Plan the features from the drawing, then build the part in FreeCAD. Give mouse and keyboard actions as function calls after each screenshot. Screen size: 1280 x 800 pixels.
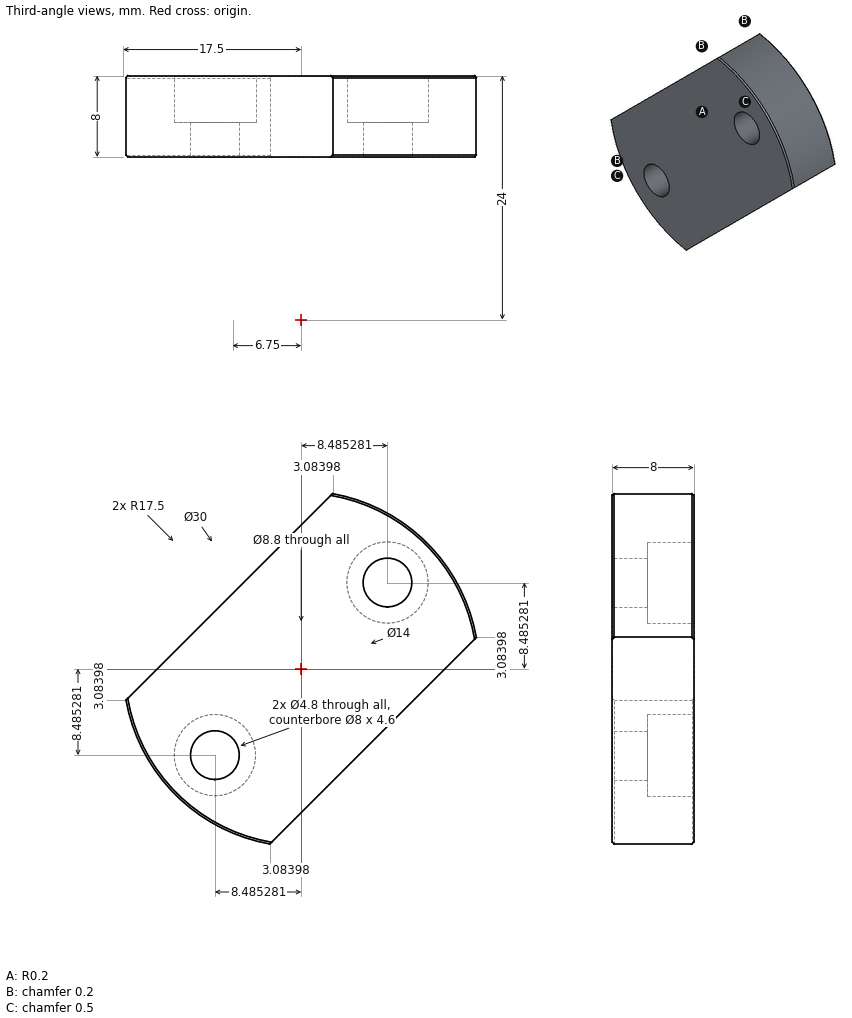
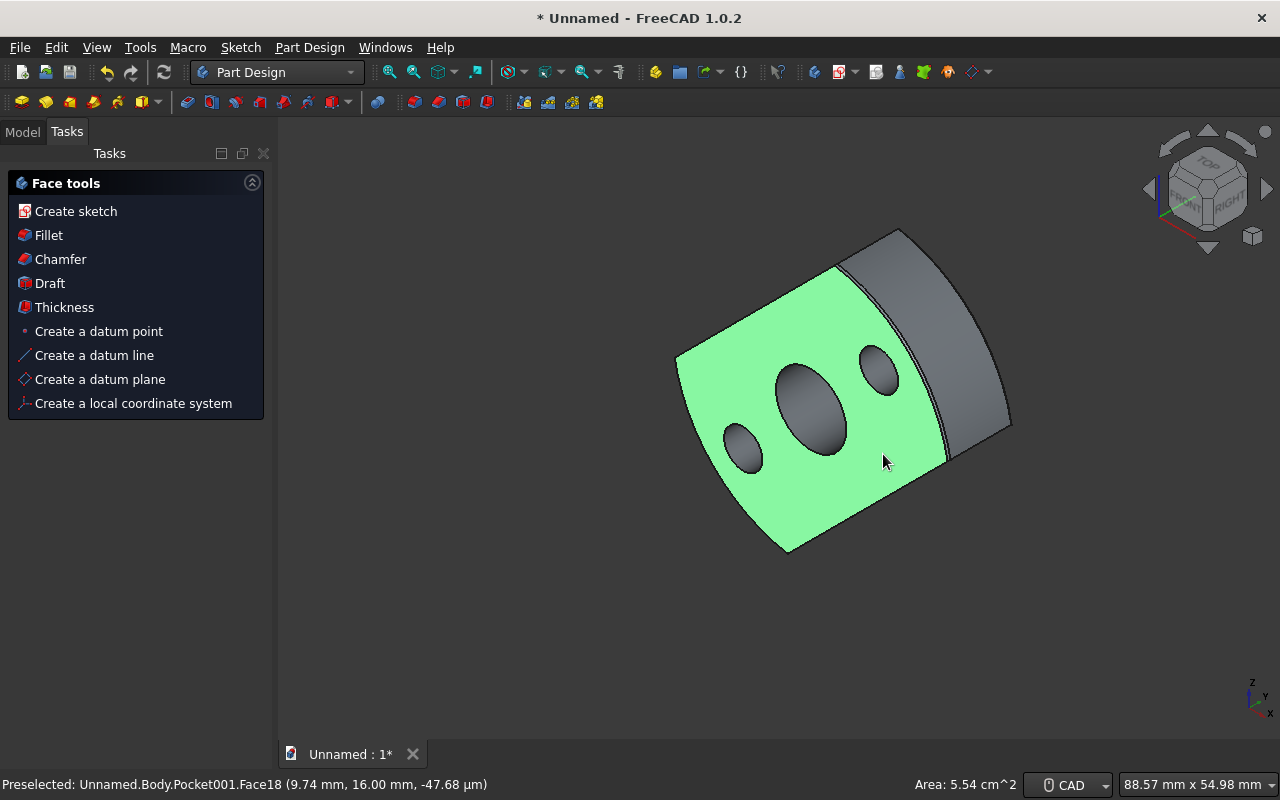
click(840, 72)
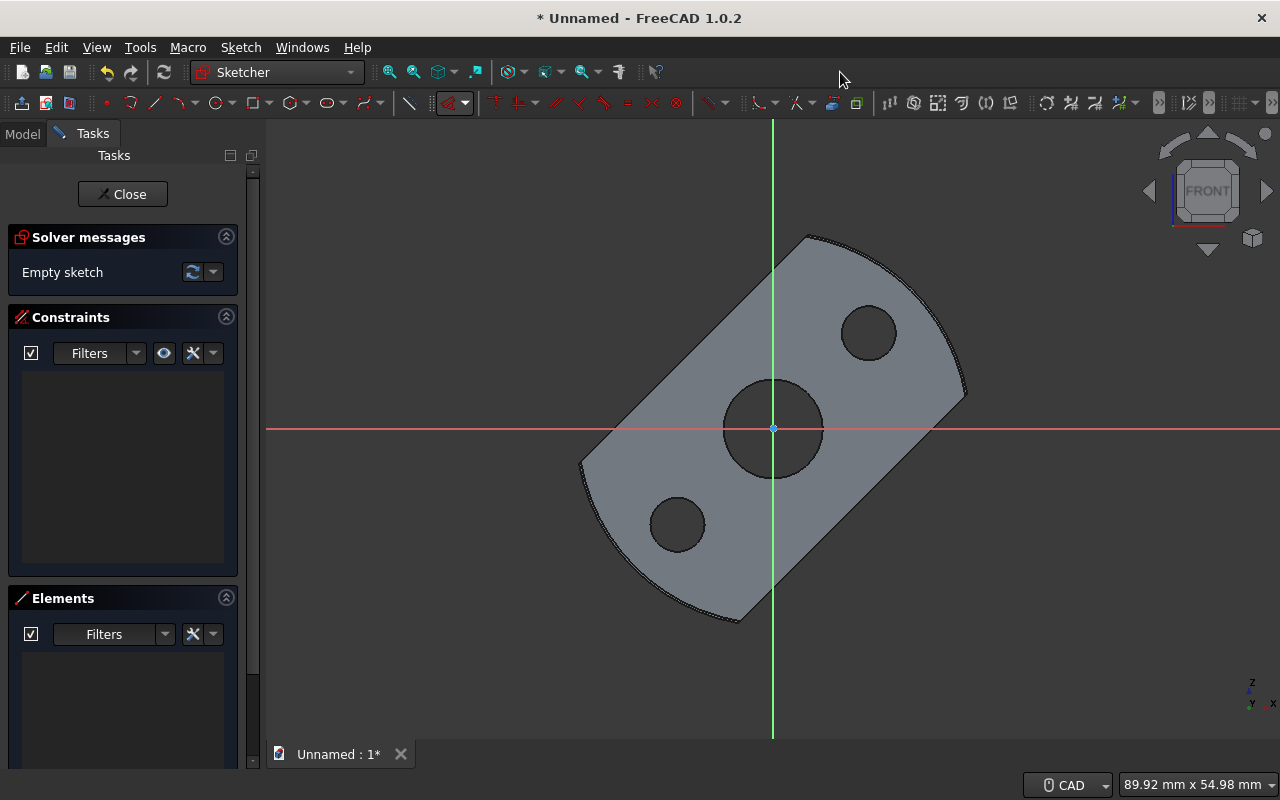
scroll(813, 429, up, 5)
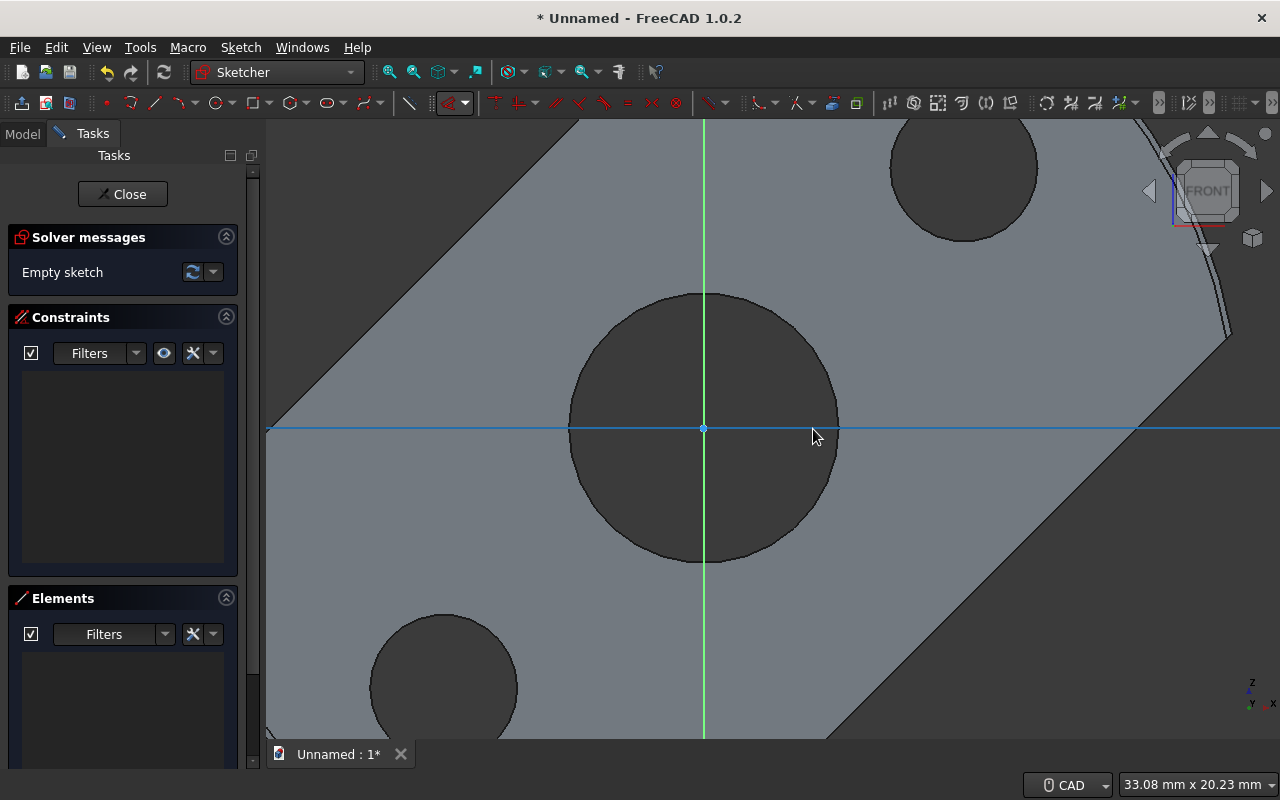
click(216, 104)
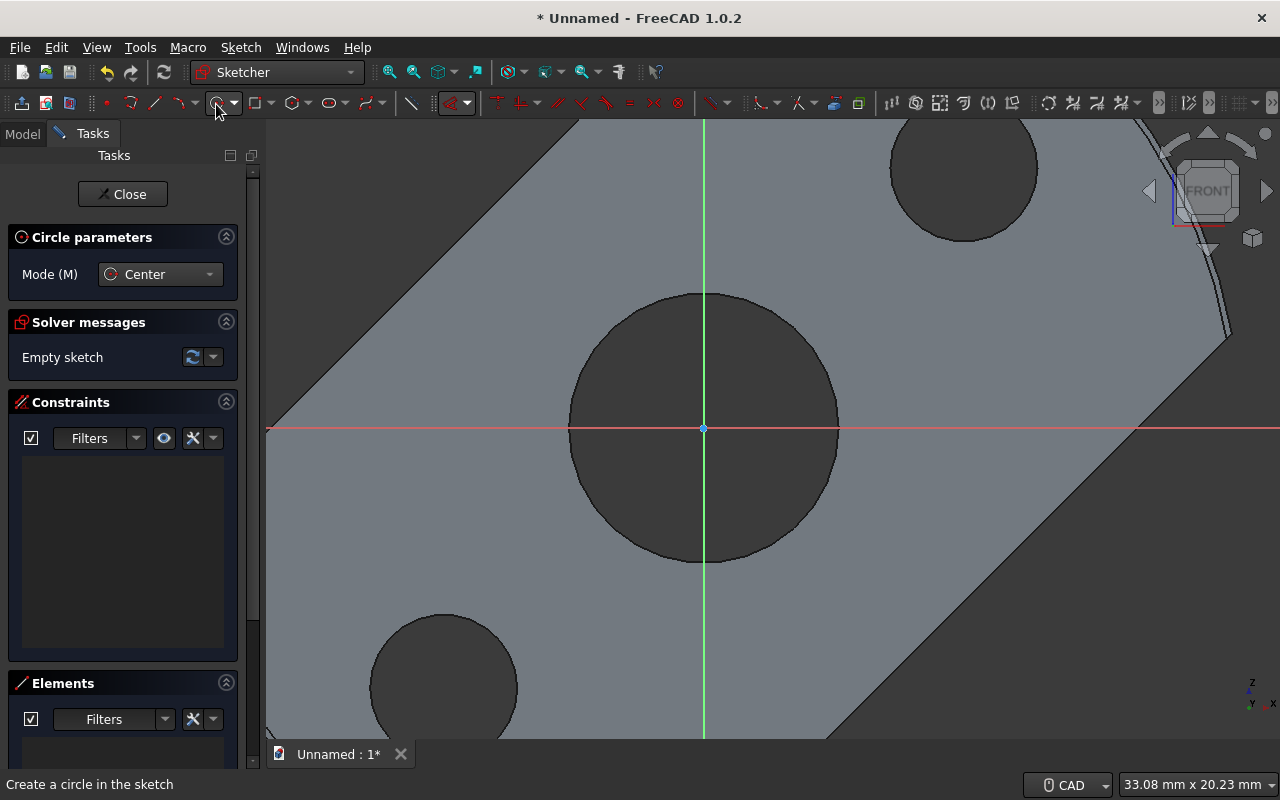
click(704, 428)
move(856, 276)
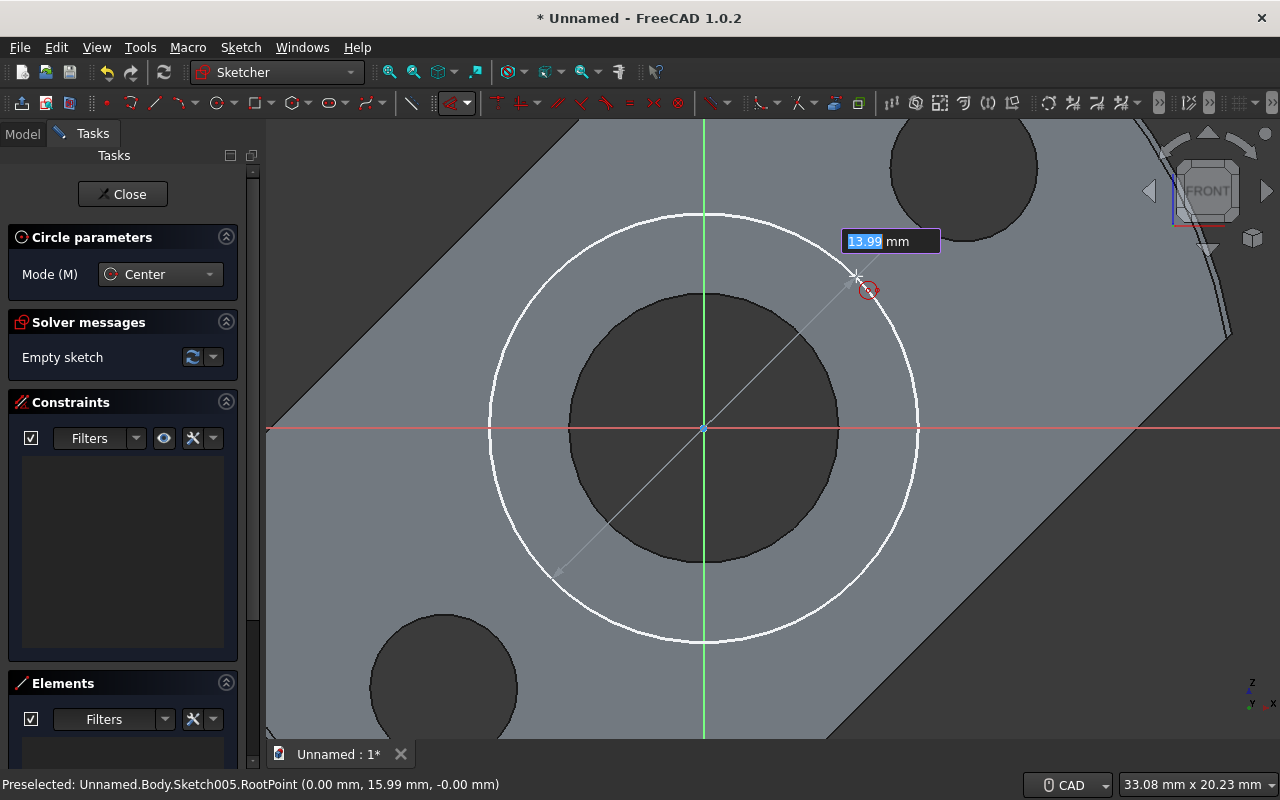
text(14)
key(Return)
key(Escape)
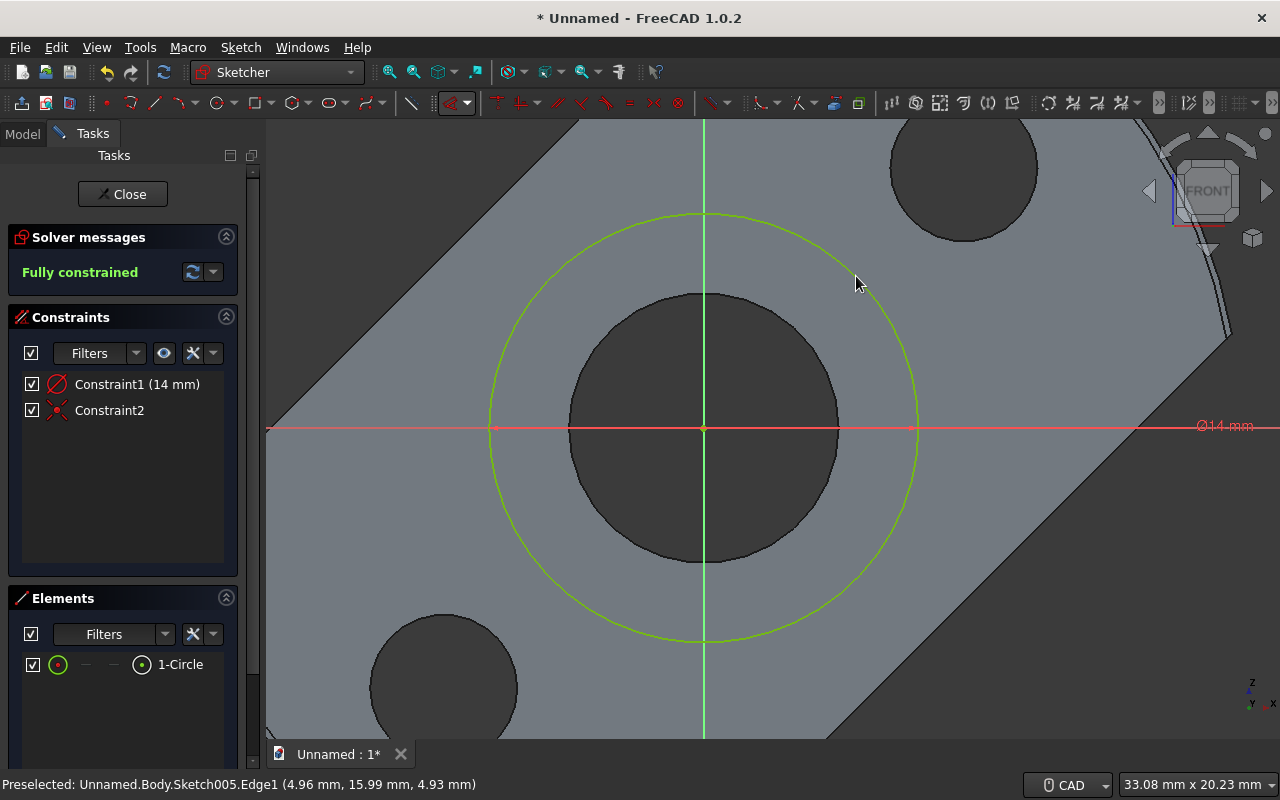
click(123, 194)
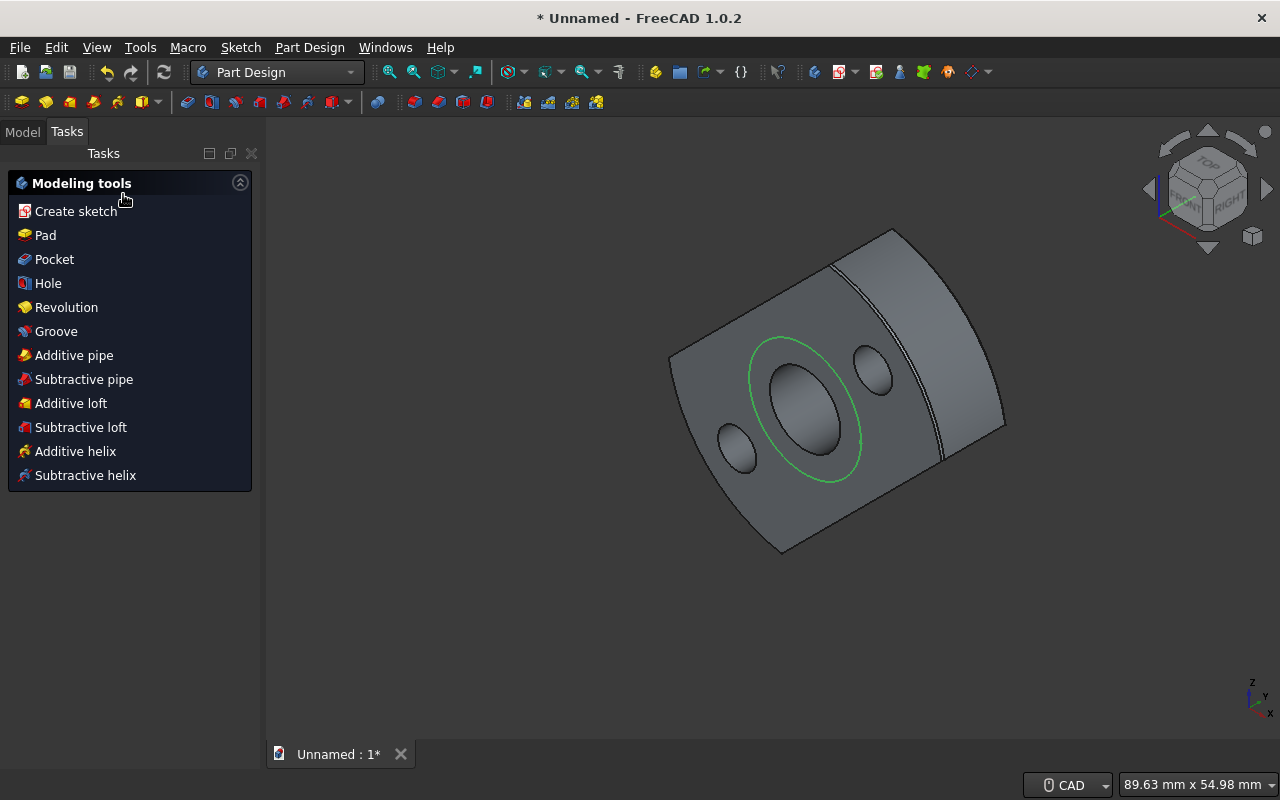
click(22, 102)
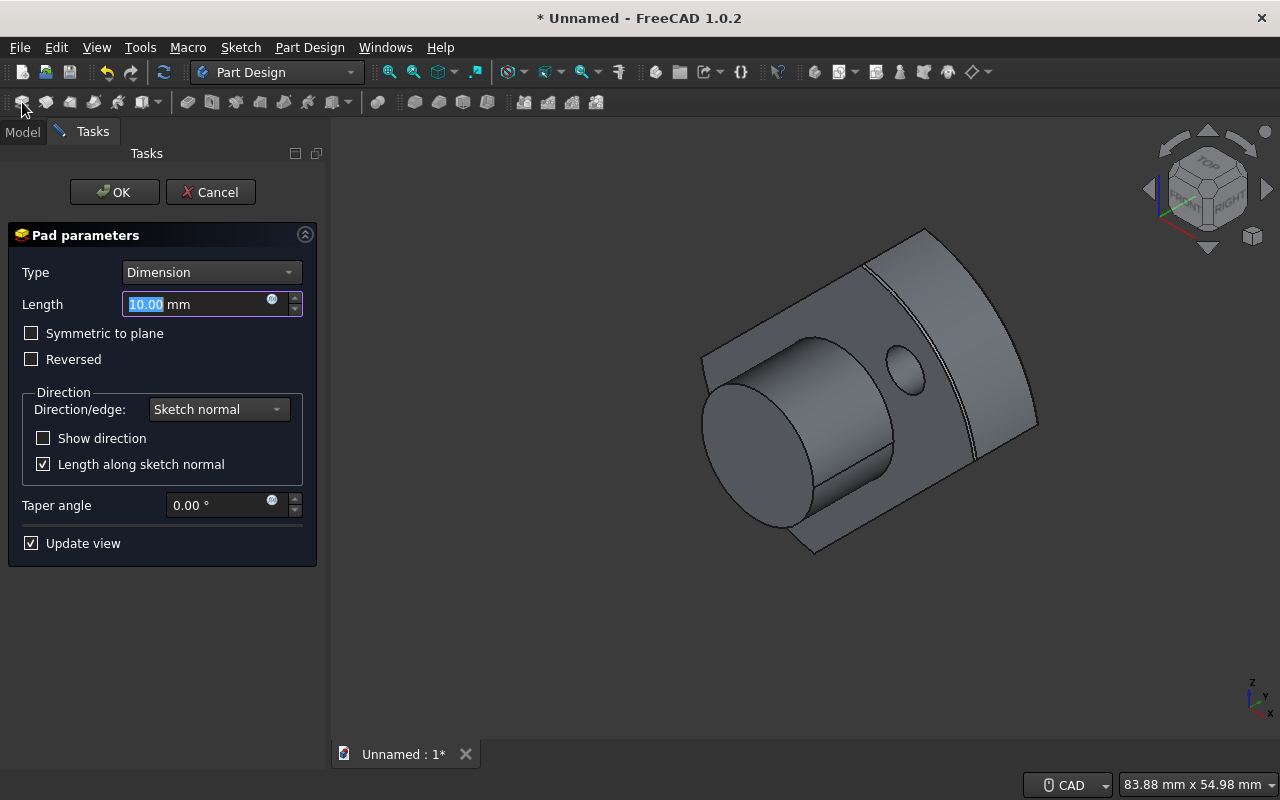
text(8)
key(Tab)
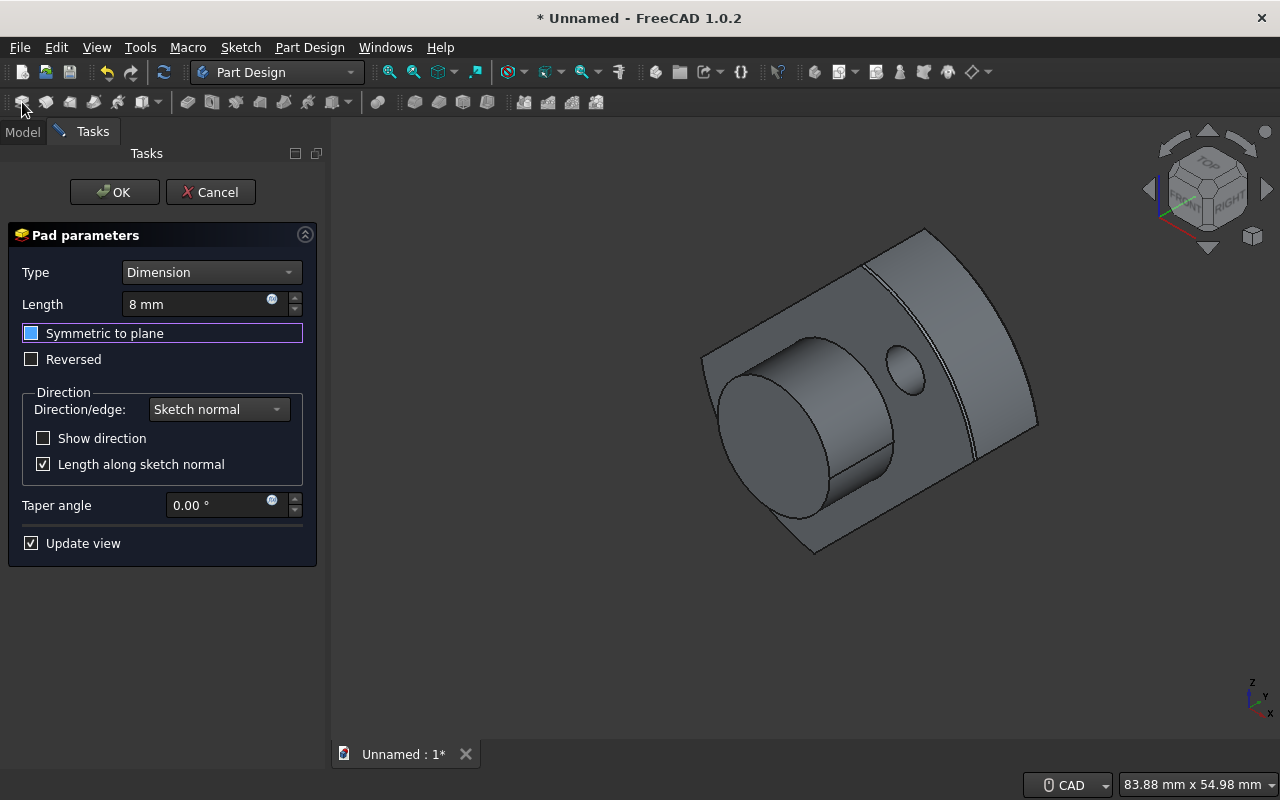
click(30, 359)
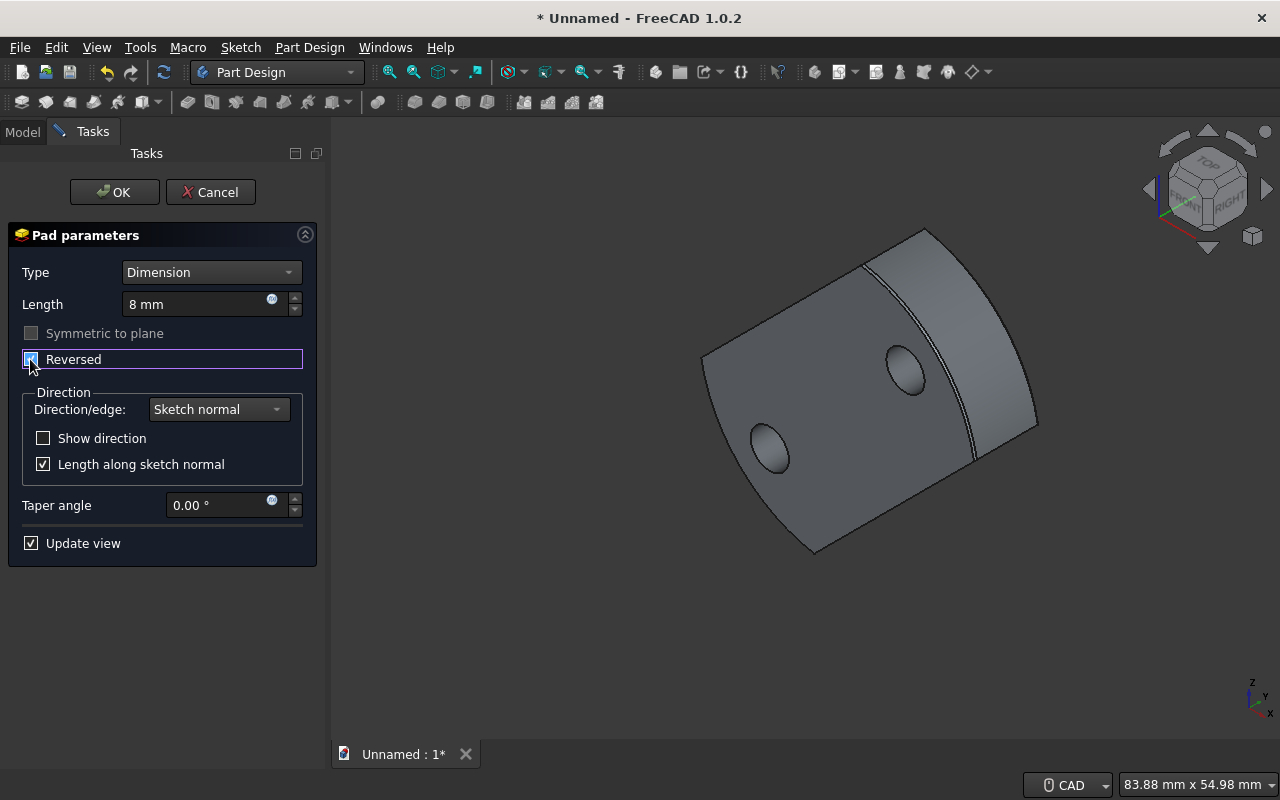
click(115, 192)